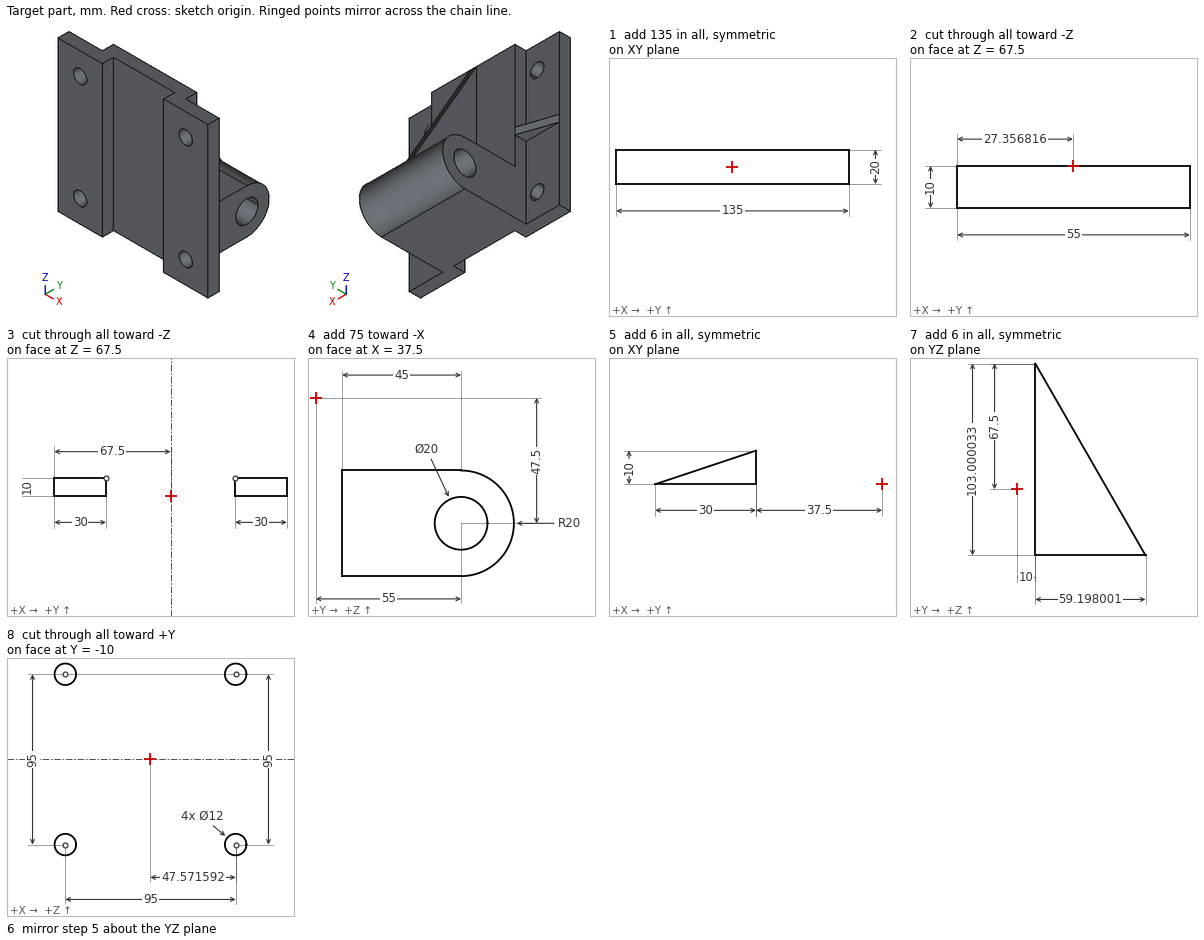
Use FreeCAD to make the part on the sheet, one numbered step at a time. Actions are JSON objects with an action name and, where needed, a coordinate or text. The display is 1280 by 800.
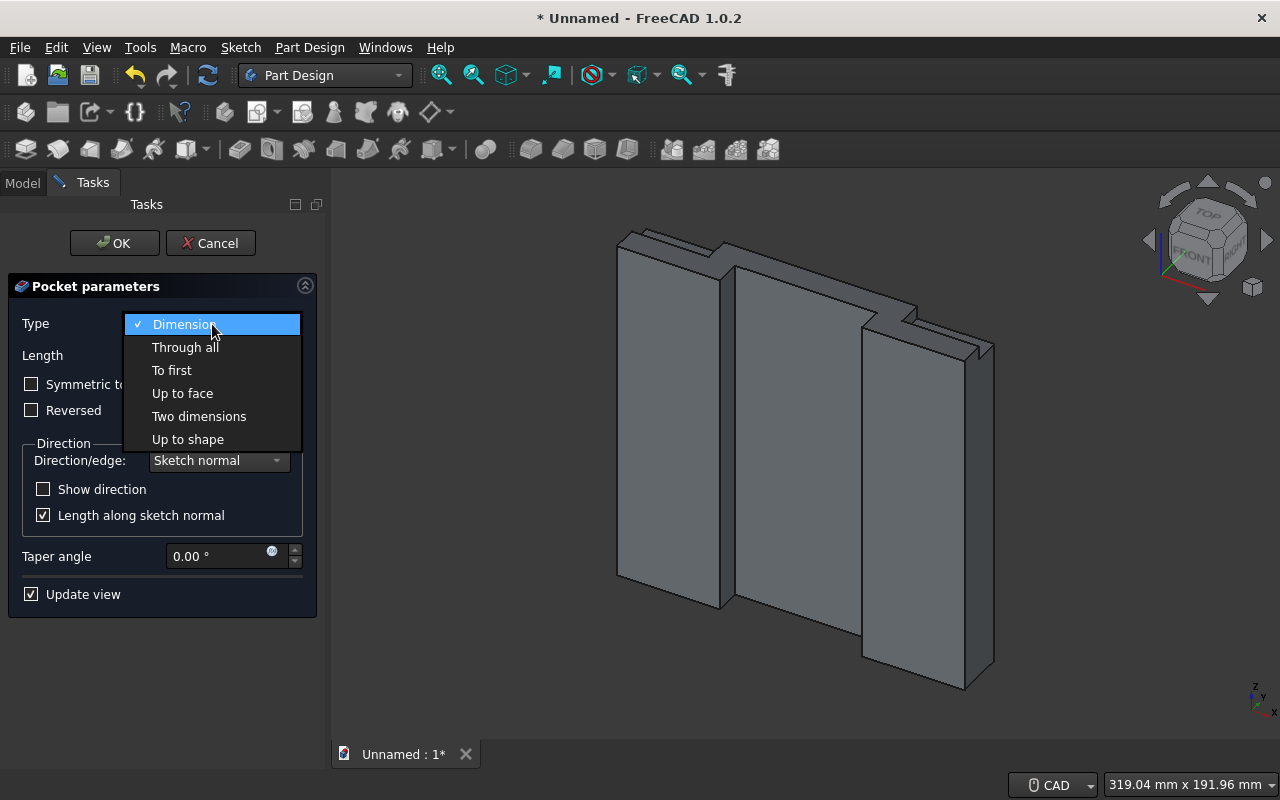
{"action": "left_click", "coordinate": [212, 348]}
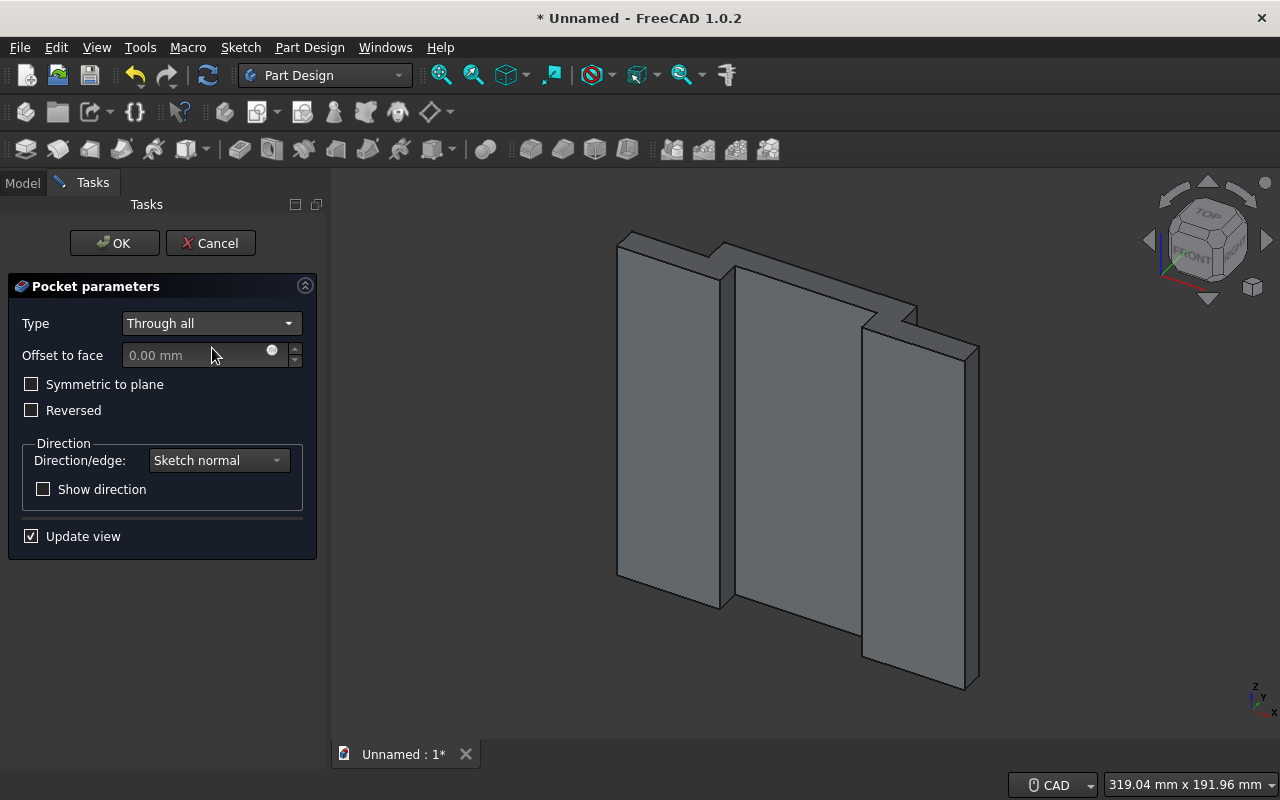
{"action": "left_click", "coordinate": [115, 243]}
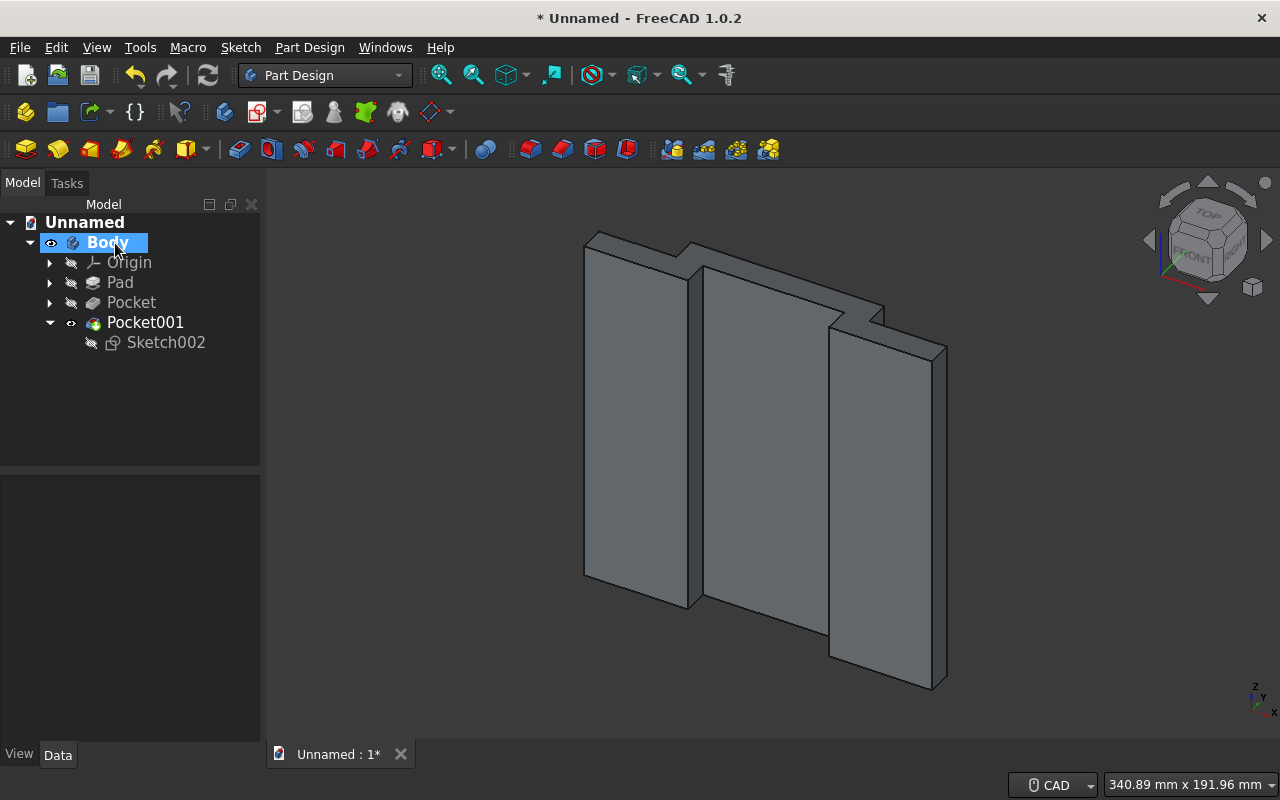
{"action": "key", "text": "0"}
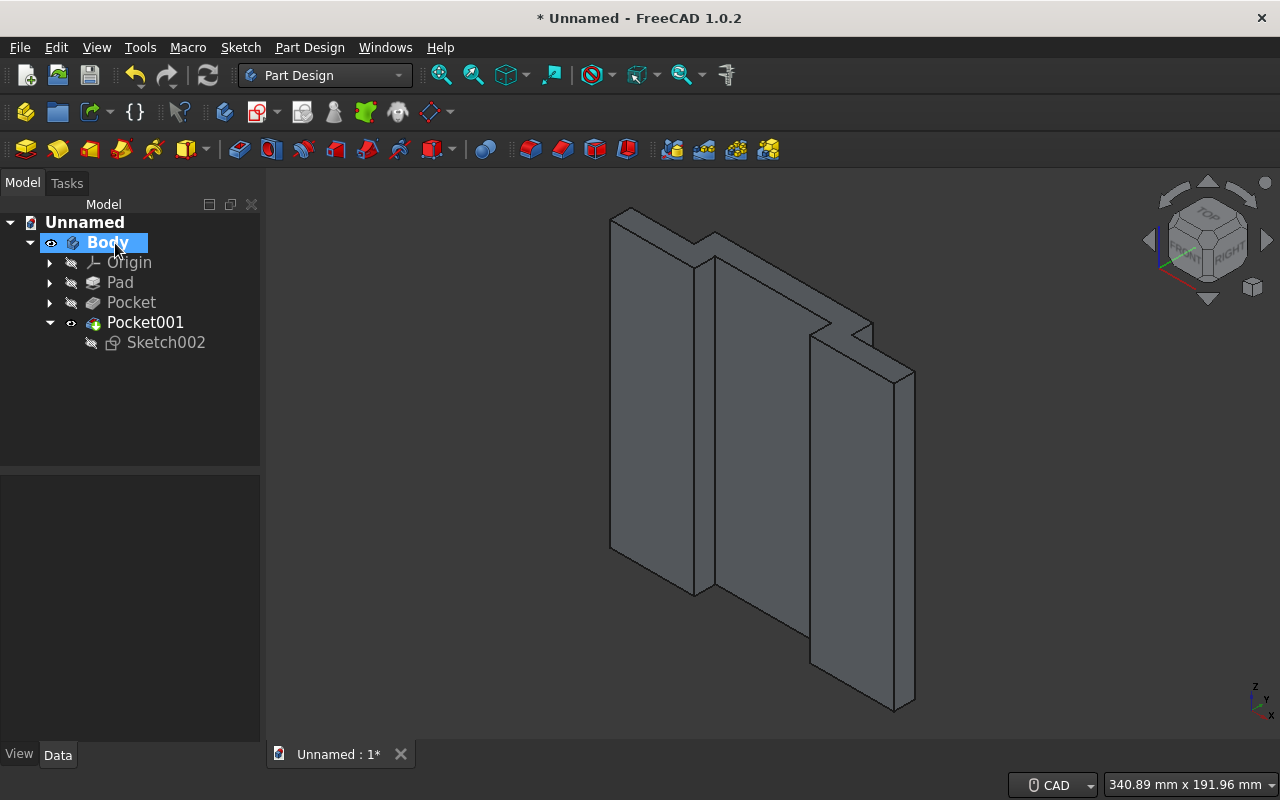
{"action": "key", "text": "3"}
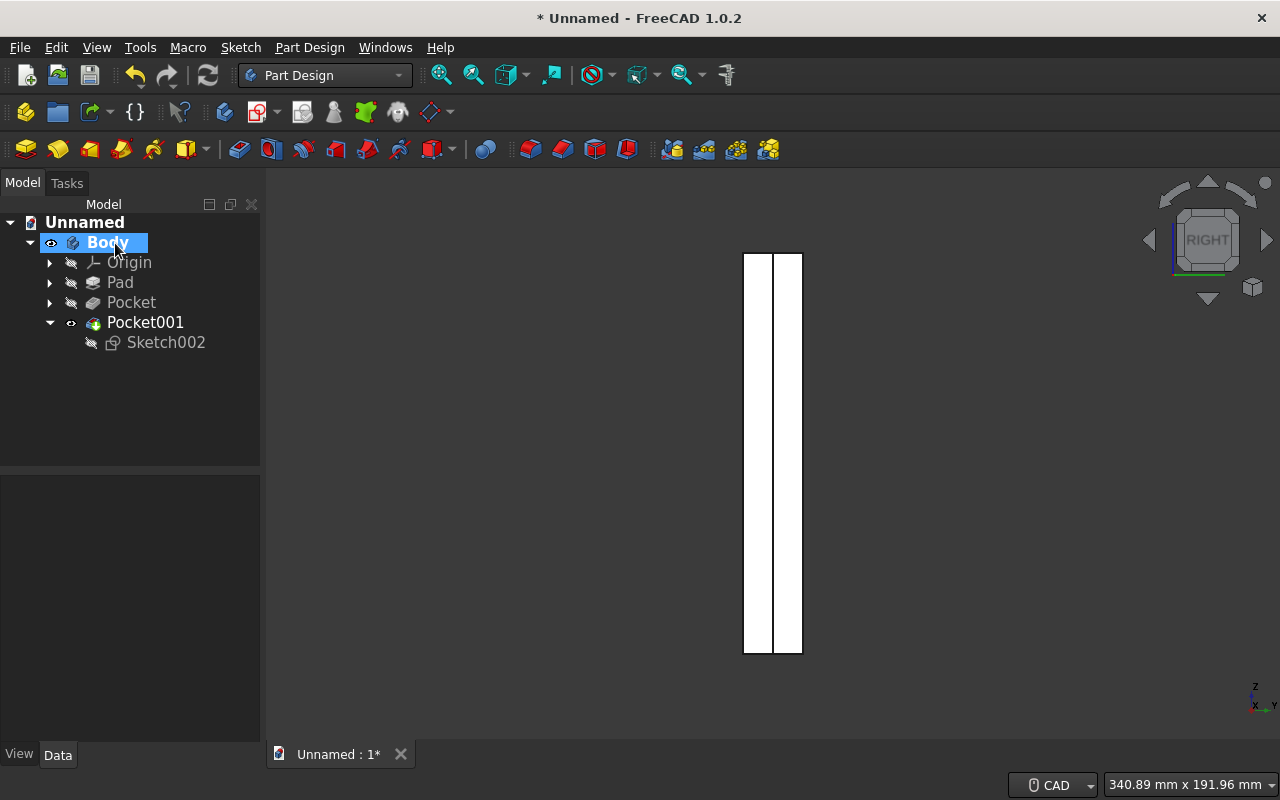
{"action": "left_click", "coordinate": [788, 280]}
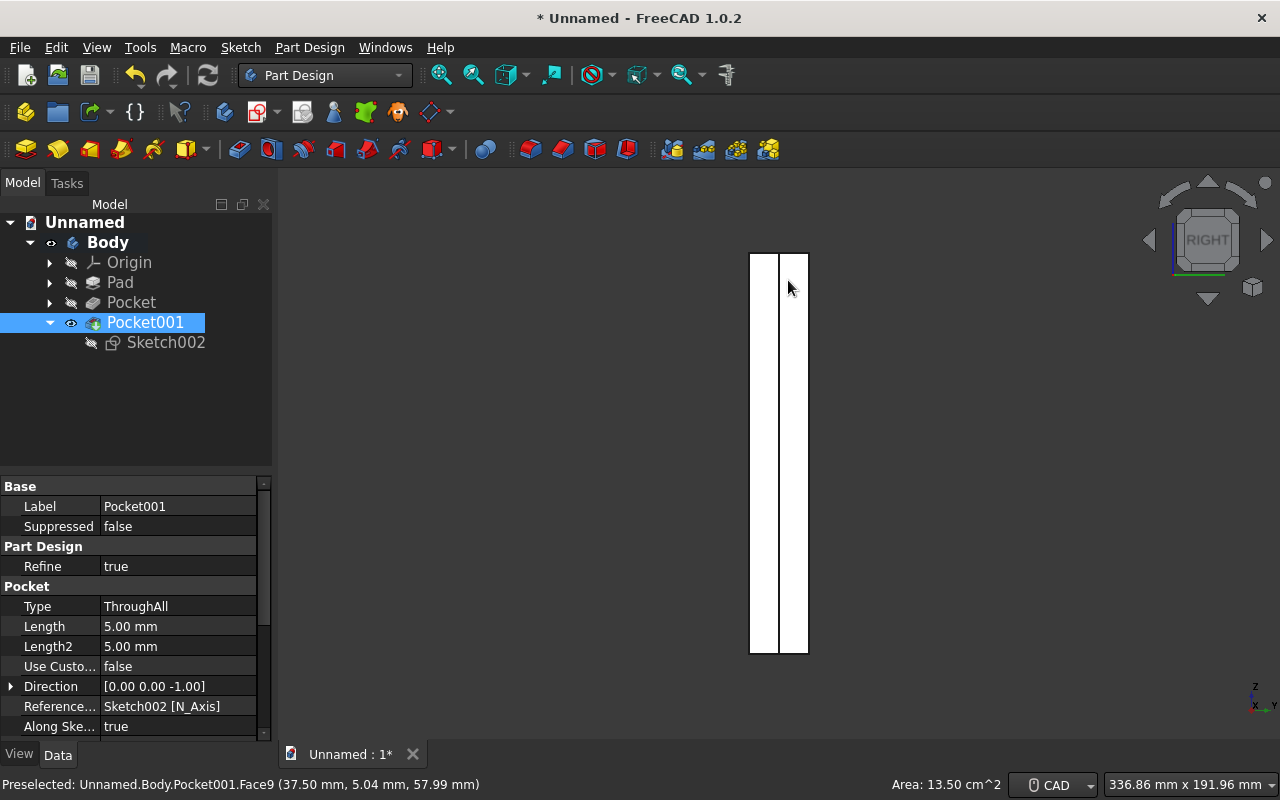
{"action": "left_click", "coordinate": [258, 112]}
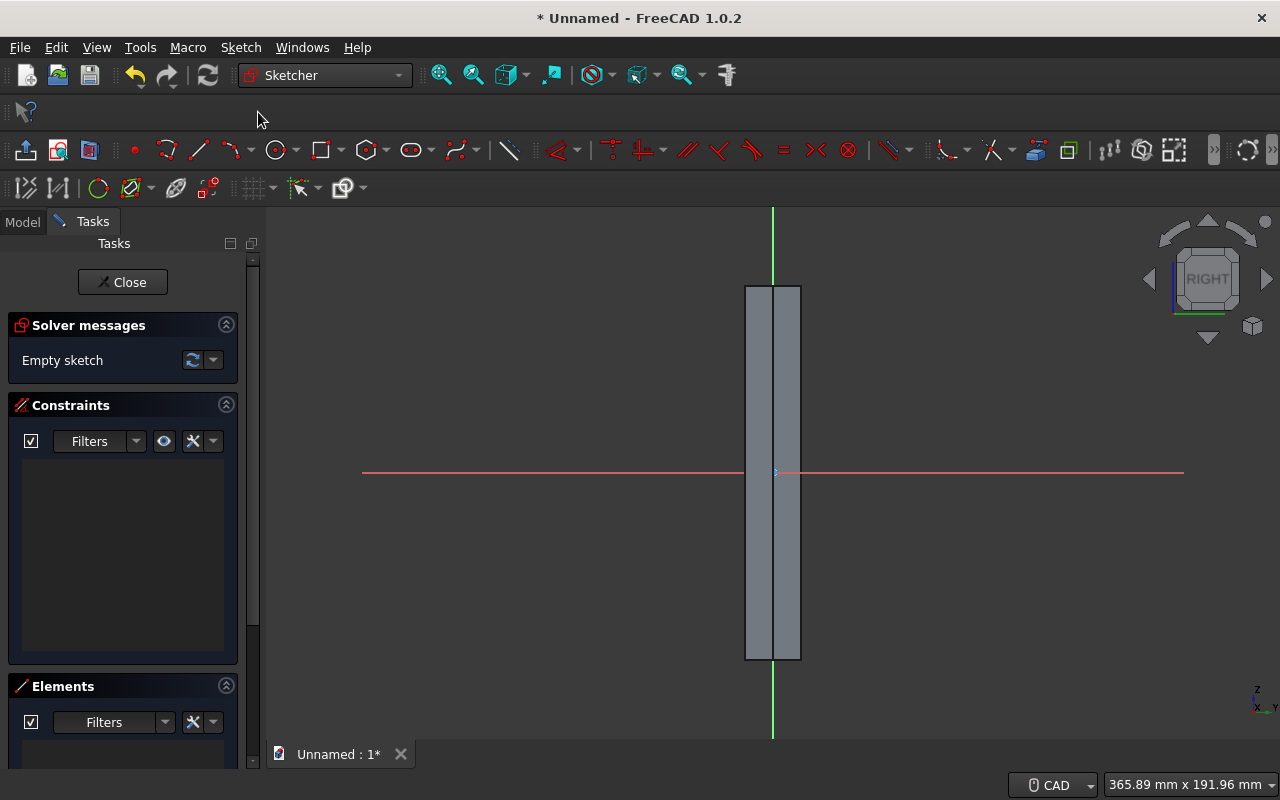
{"action": "left_click", "coordinate": [90, 150]}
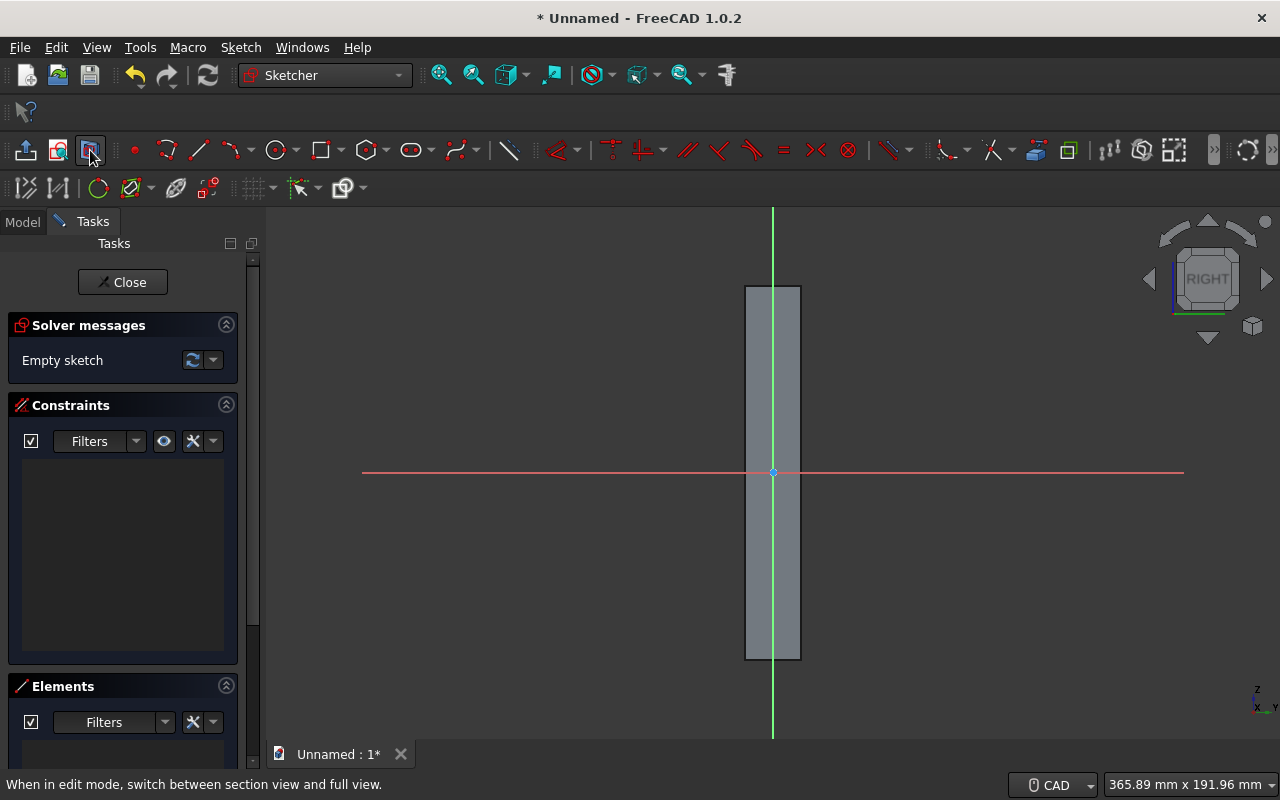
{"action": "scroll", "coordinate": [1087, 680], "scroll_direction": "up", "scroll_amount": 3}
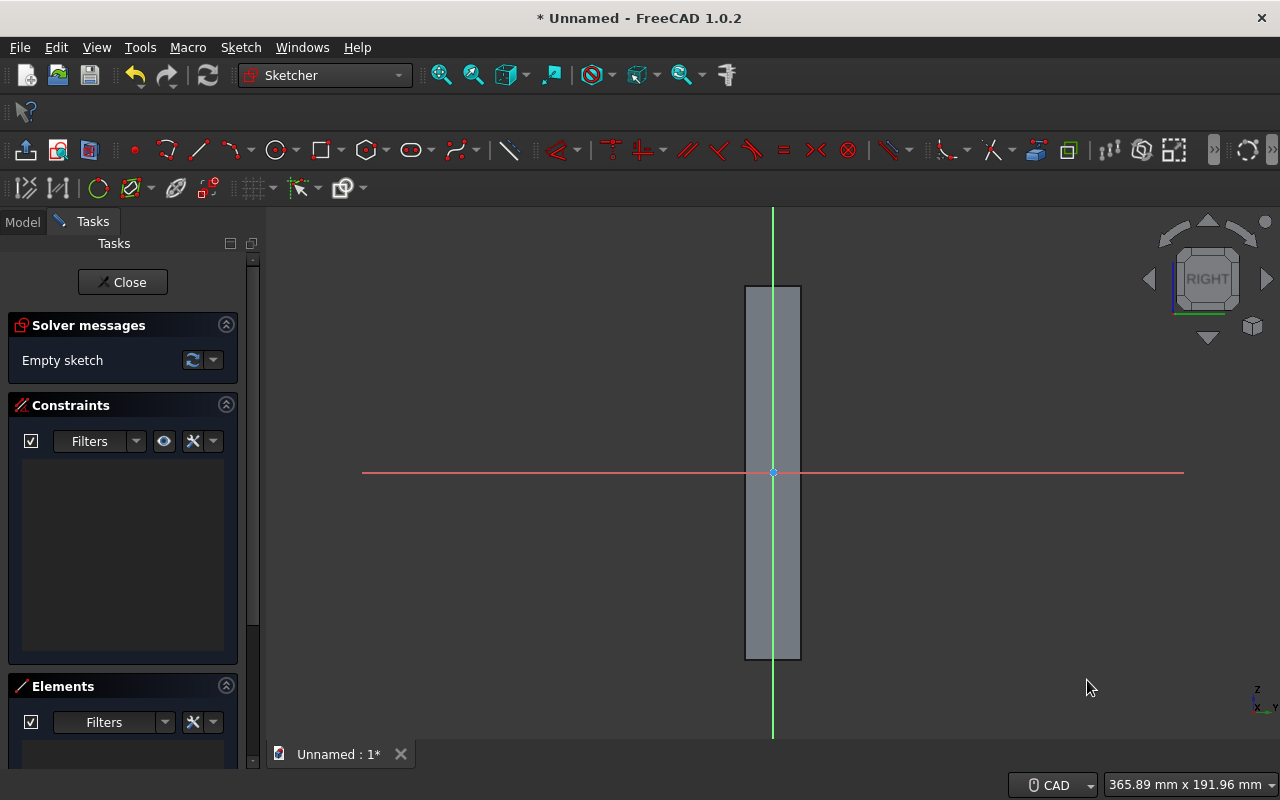
{"action": "key", "text": "g m"}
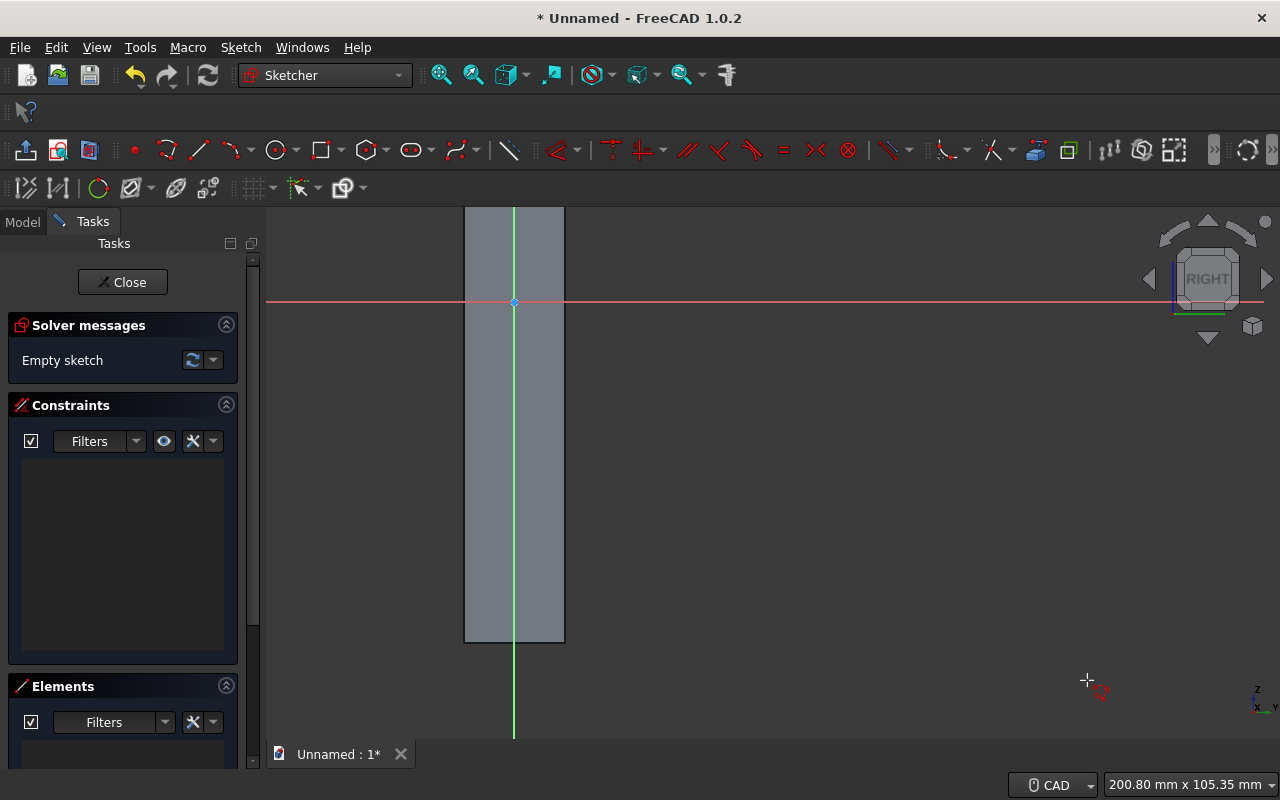
{"action": "left_click", "coordinate": [792, 441]}
{"action": "left_click", "coordinate": [565, 441]}
{"action": "left_click", "coordinate": [565, 643]}
{"action": "left_click", "coordinate": [792, 643]}
{"action": "right_click", "coordinate": [792, 643]}